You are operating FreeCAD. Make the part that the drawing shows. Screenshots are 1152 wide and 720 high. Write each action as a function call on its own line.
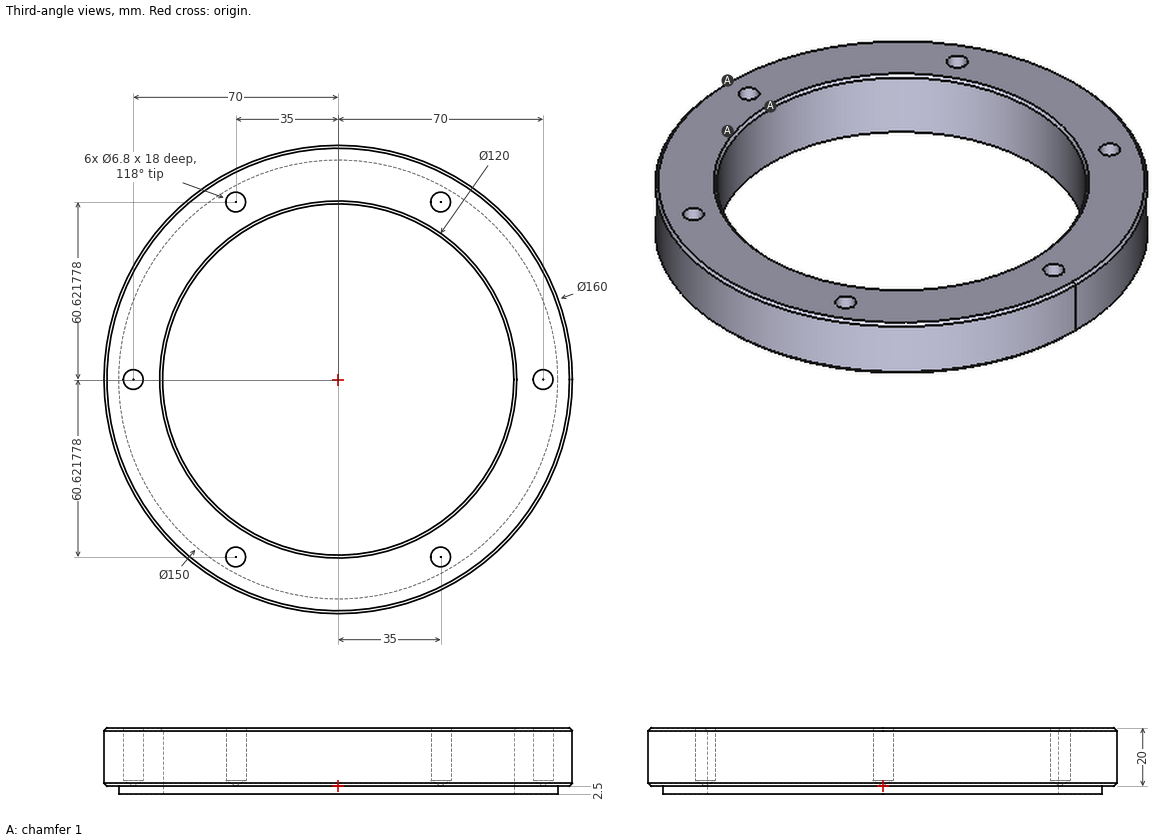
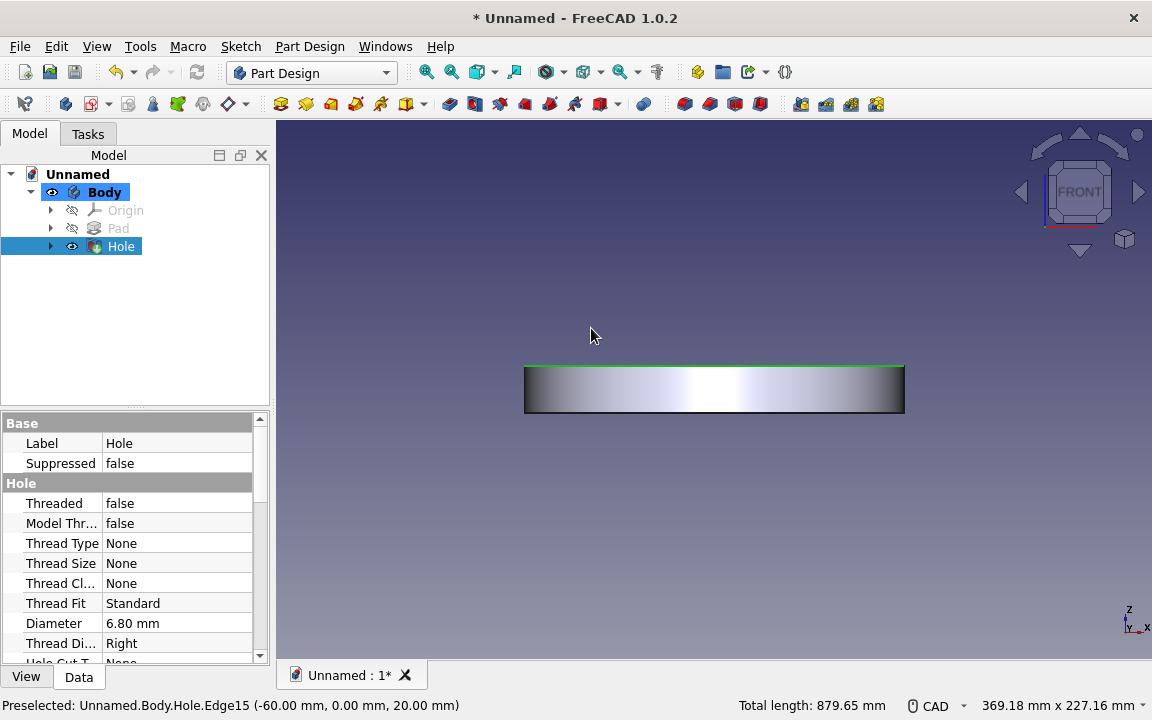
click(427, 72)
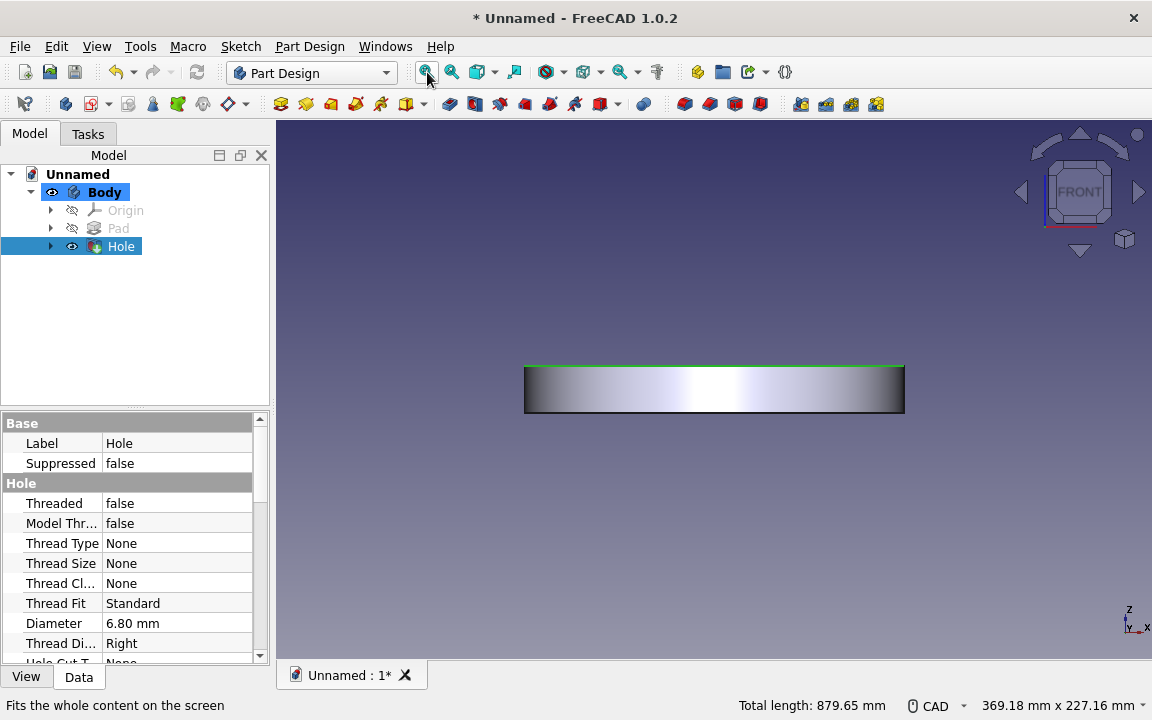
click(560, 412, ctrl)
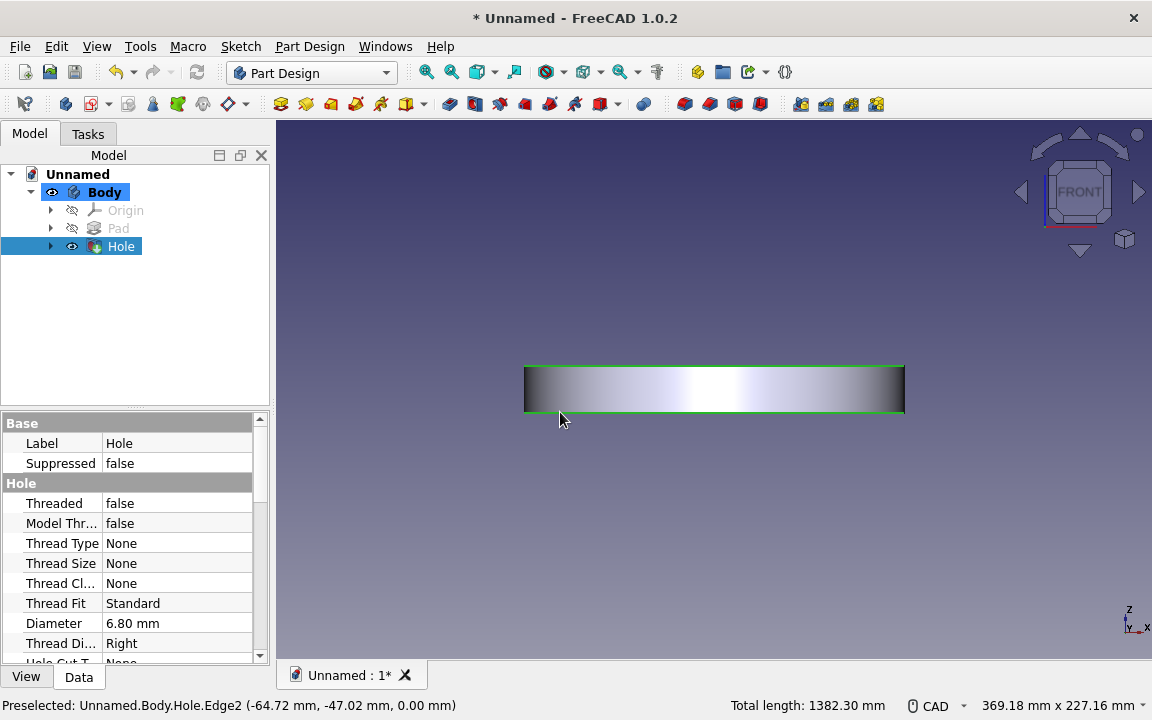
click(710, 104)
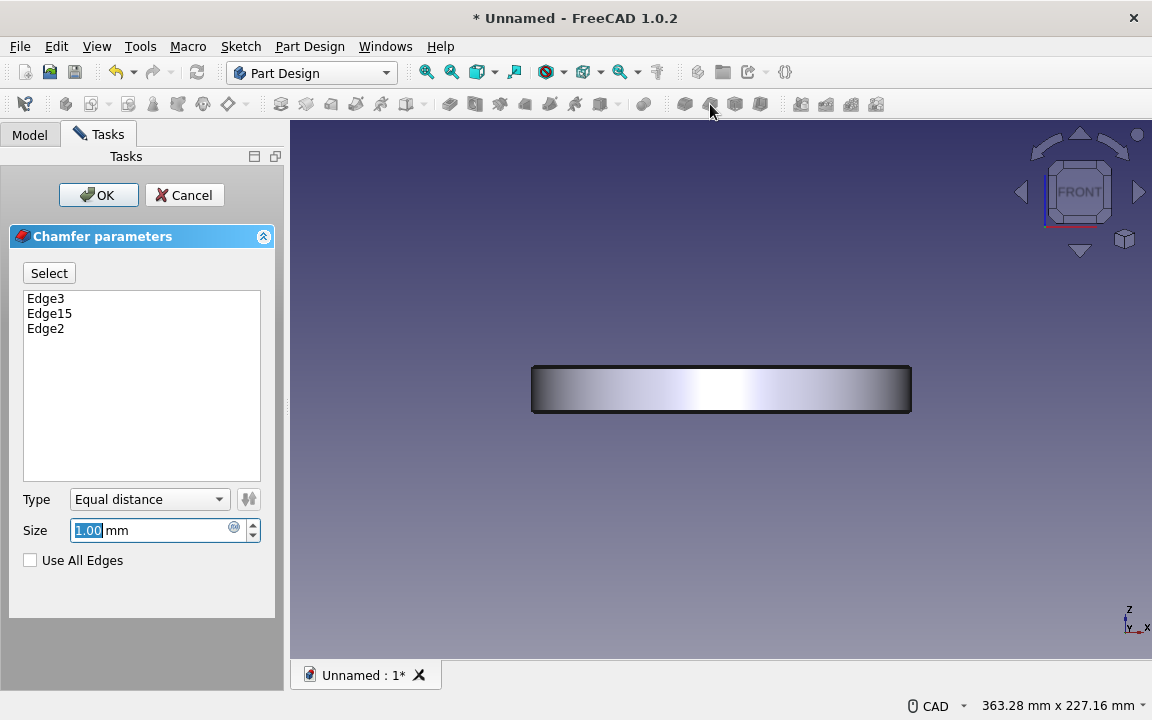
text(1)
key(Tab)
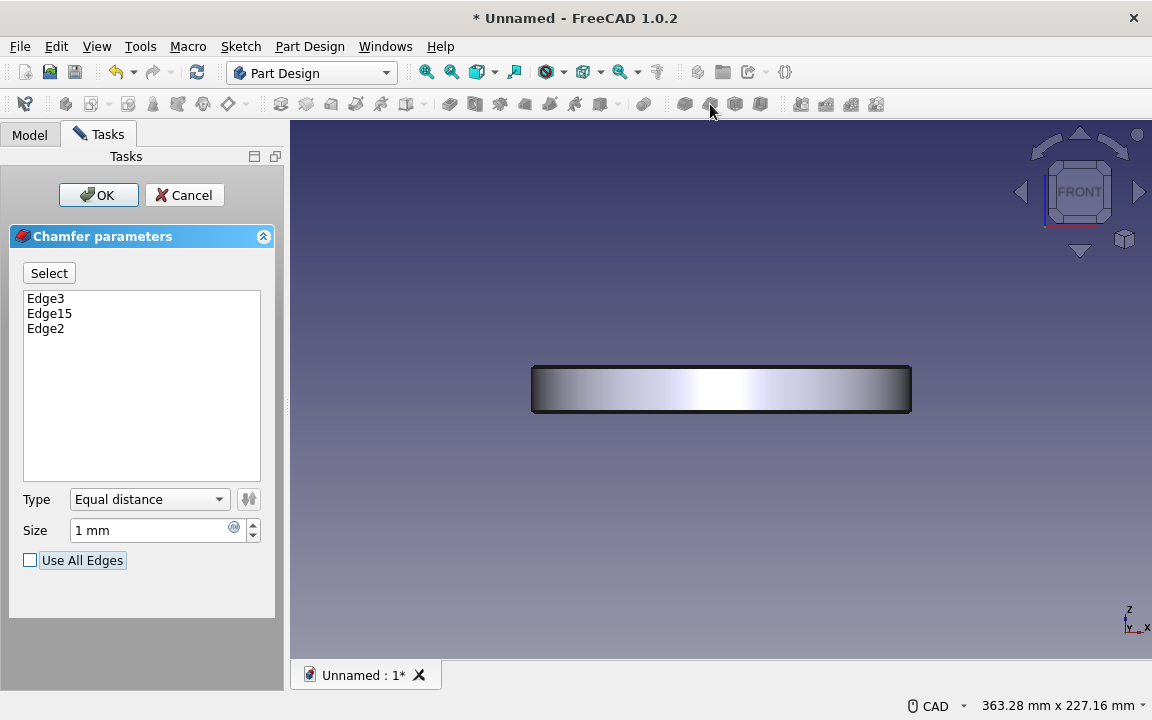
click(99, 195)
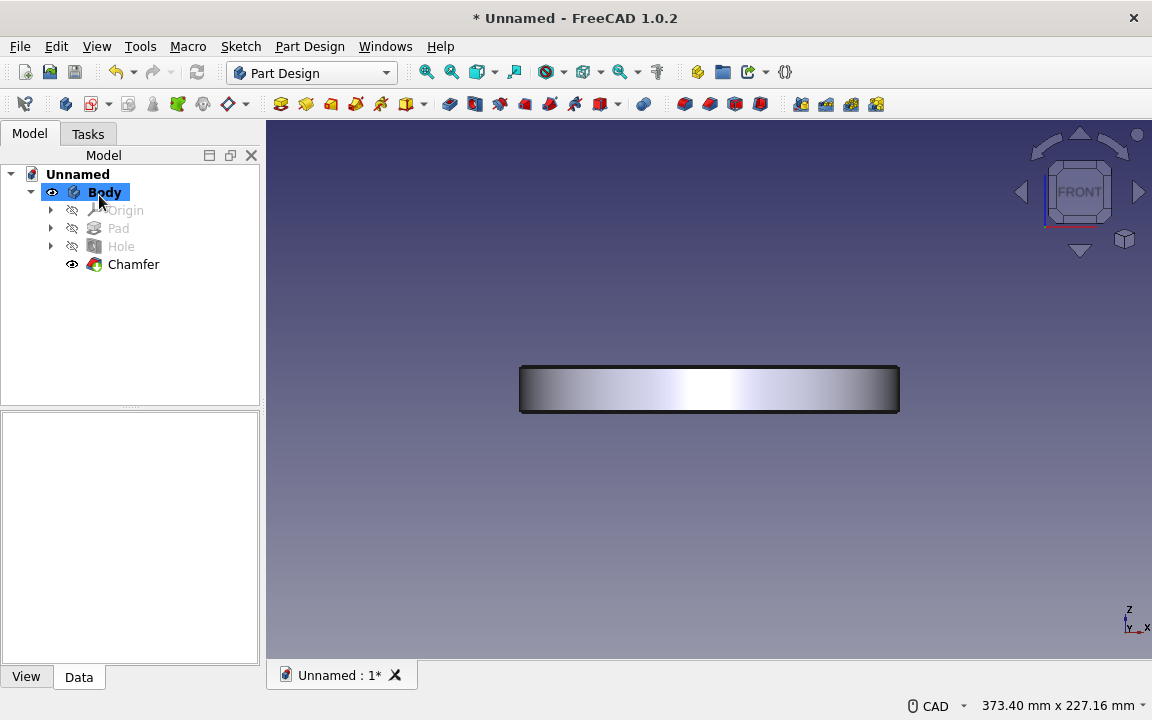
key(v)
key(f)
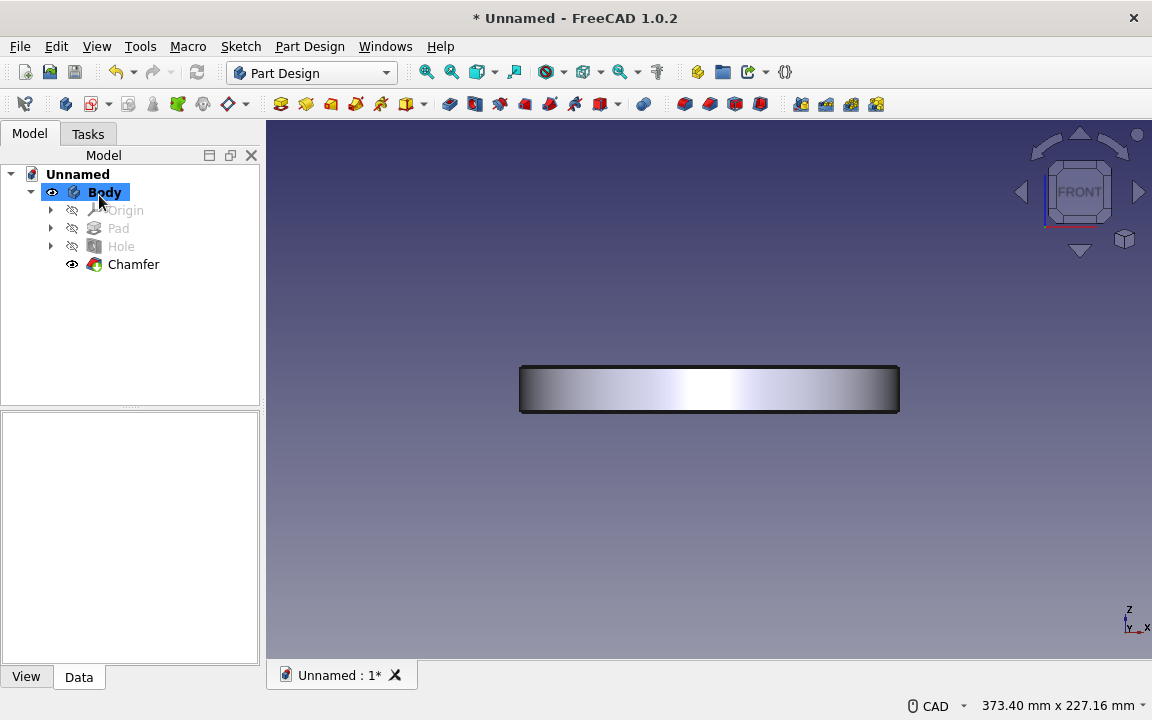
click(51, 210)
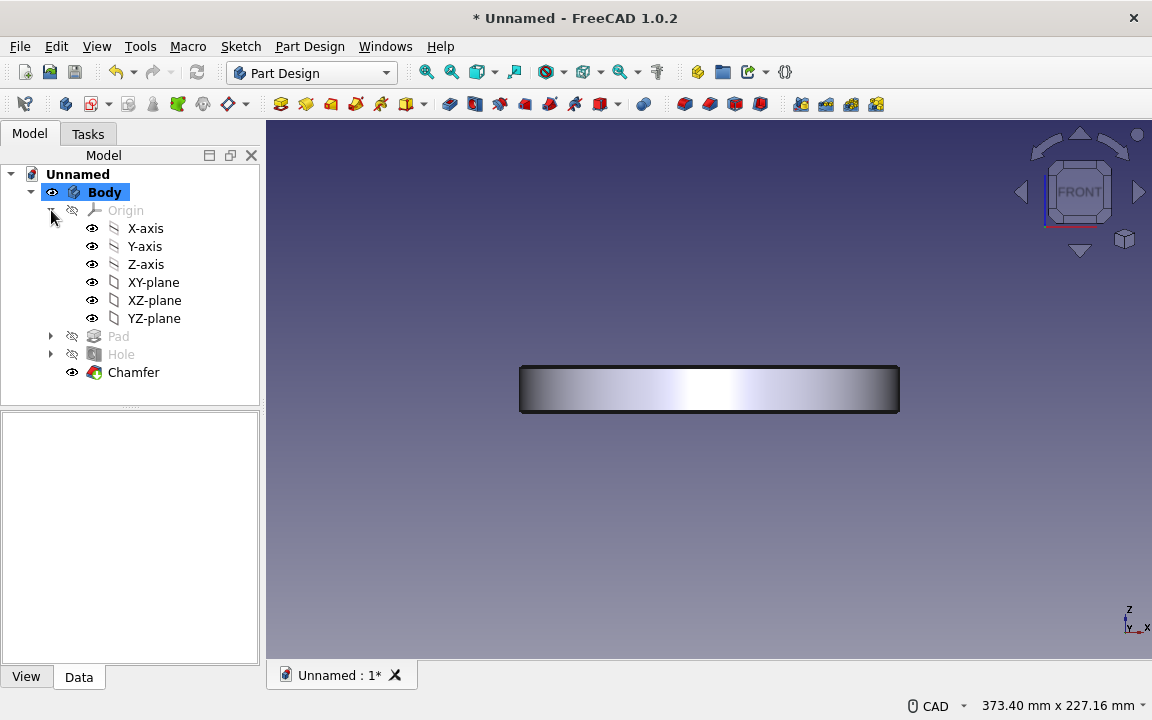
click(137, 282)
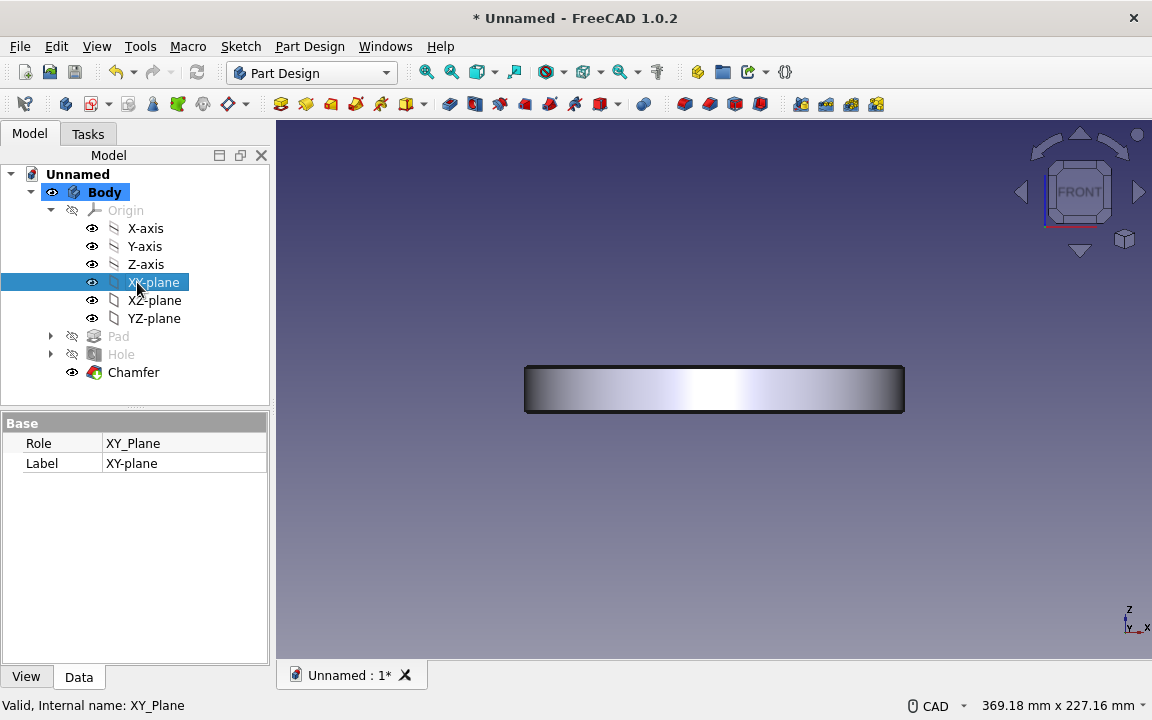
click(228, 104)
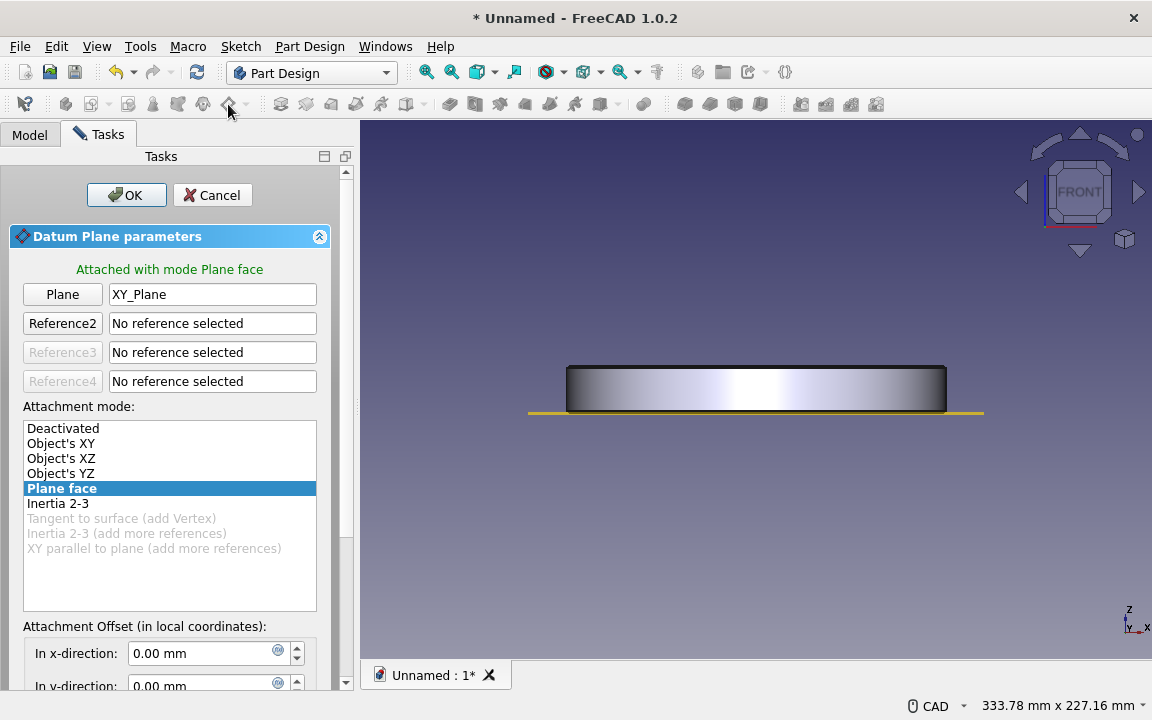
scroll(346, 428, down, 2)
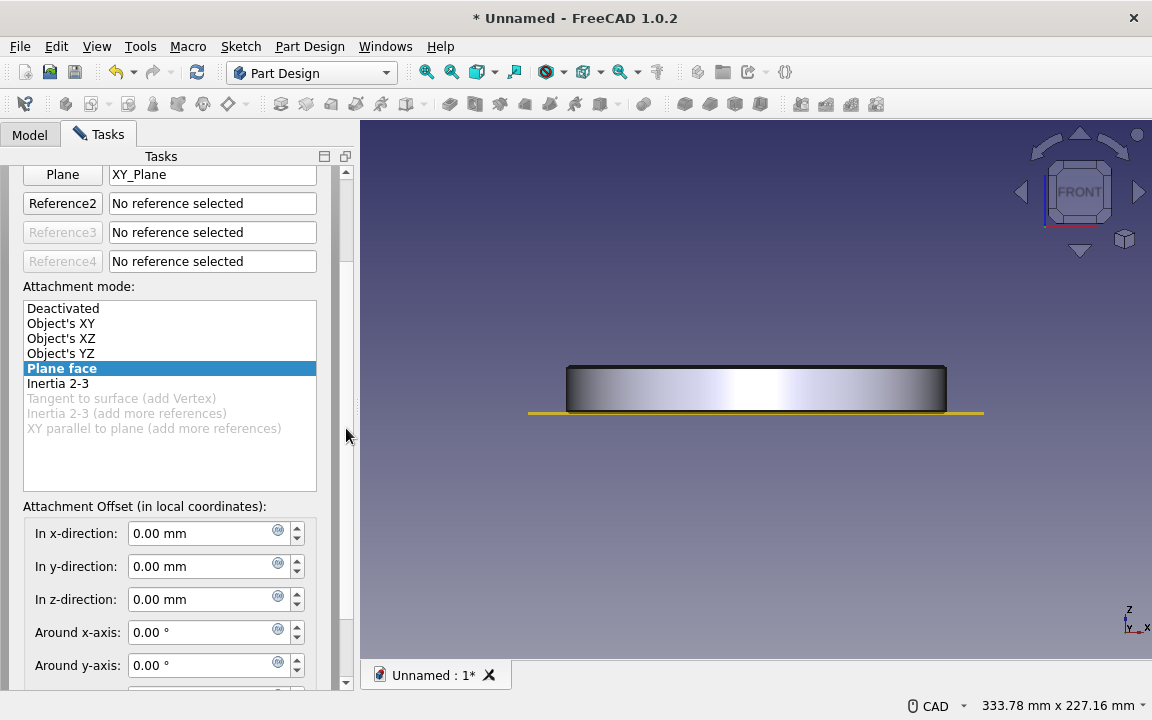
triple_click(210, 600)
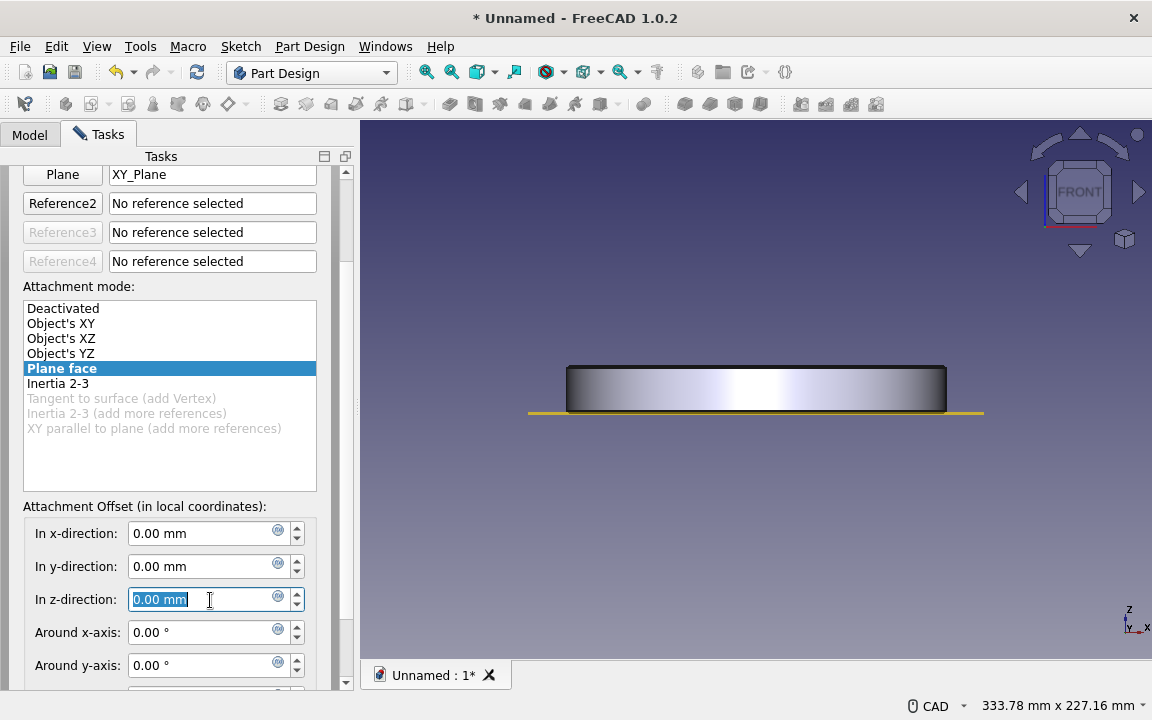
text(-2.5)
key(Tab)